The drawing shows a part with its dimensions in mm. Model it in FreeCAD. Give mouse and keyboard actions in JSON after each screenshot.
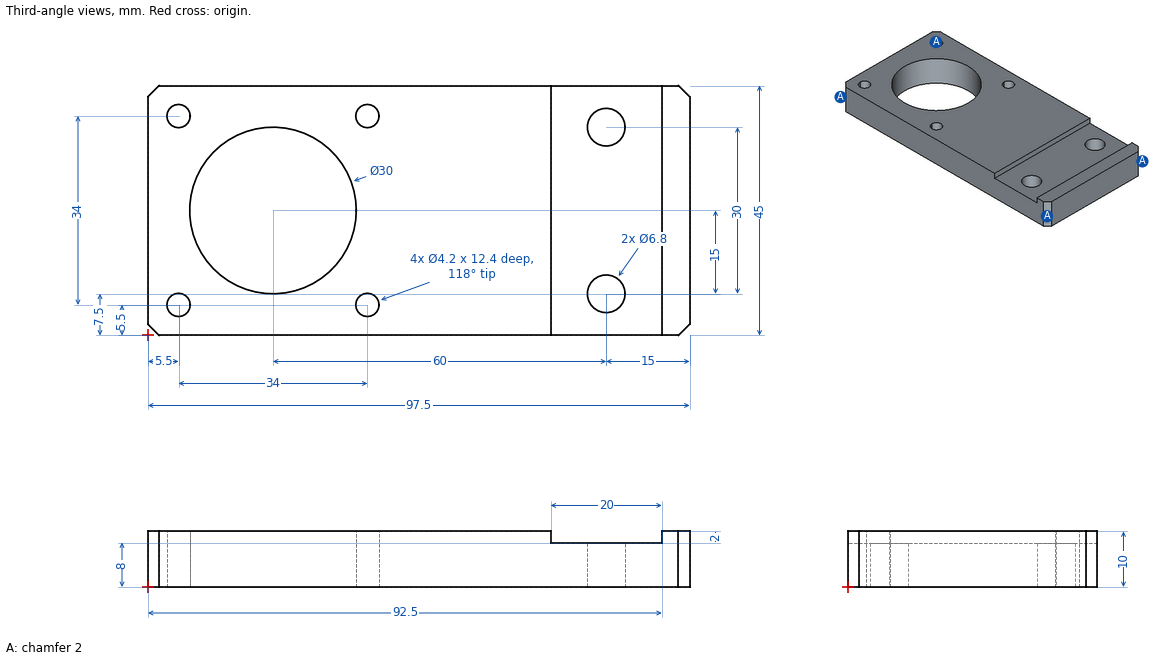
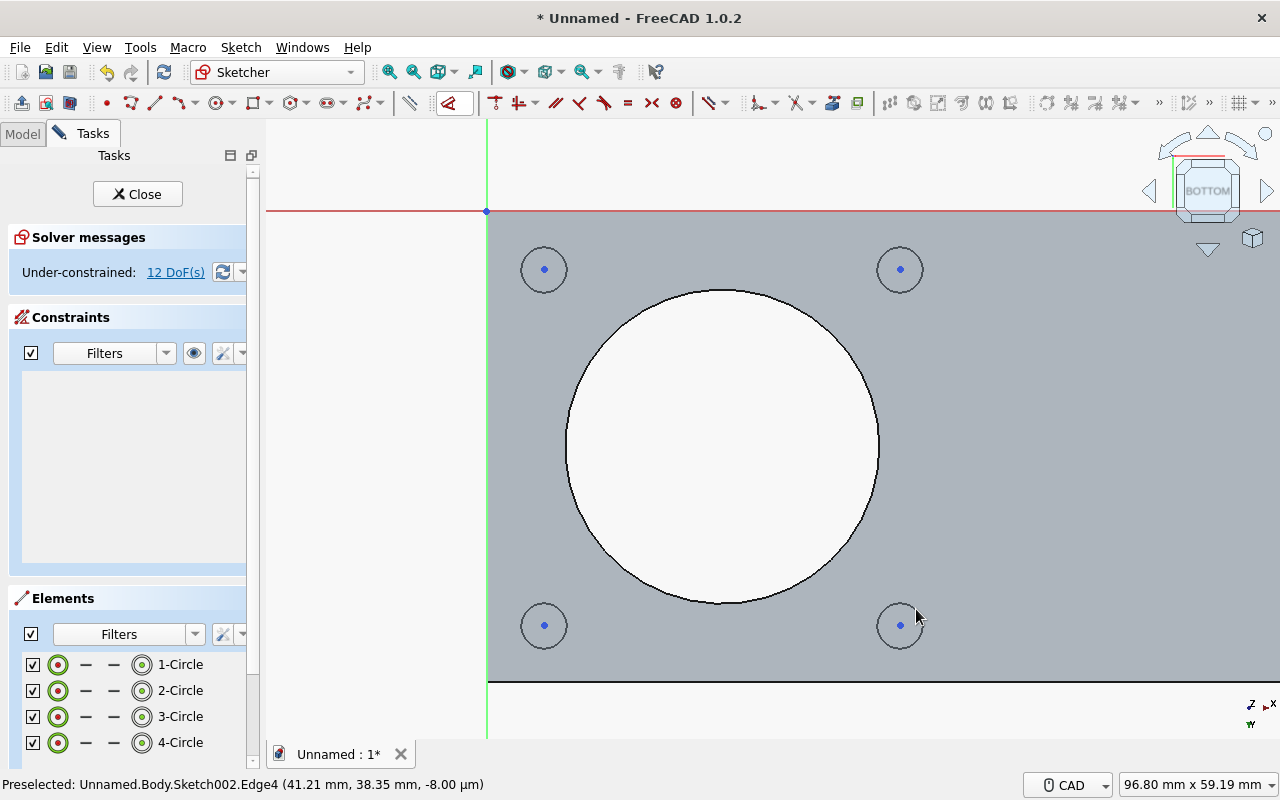
{"action": "left_click", "coordinate": [916, 254]}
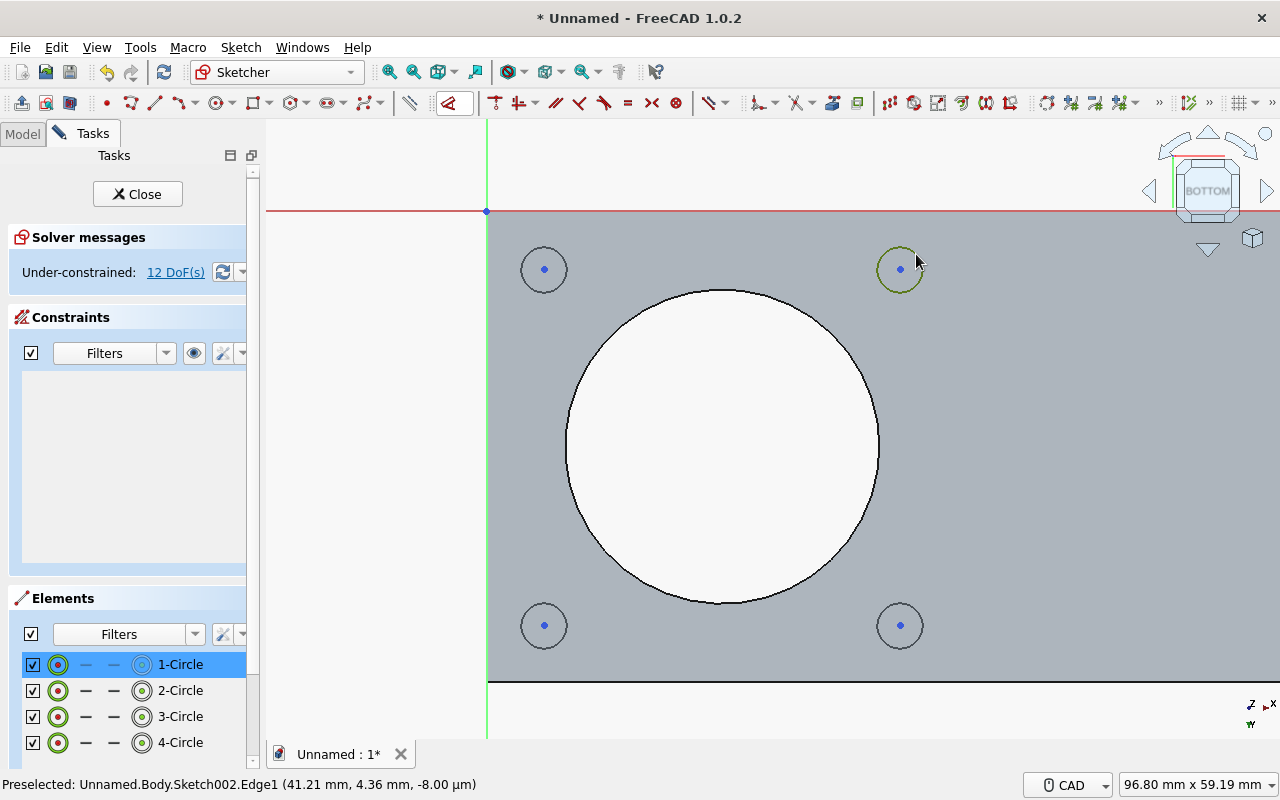
{"action": "left_click", "coordinate": [560, 254]}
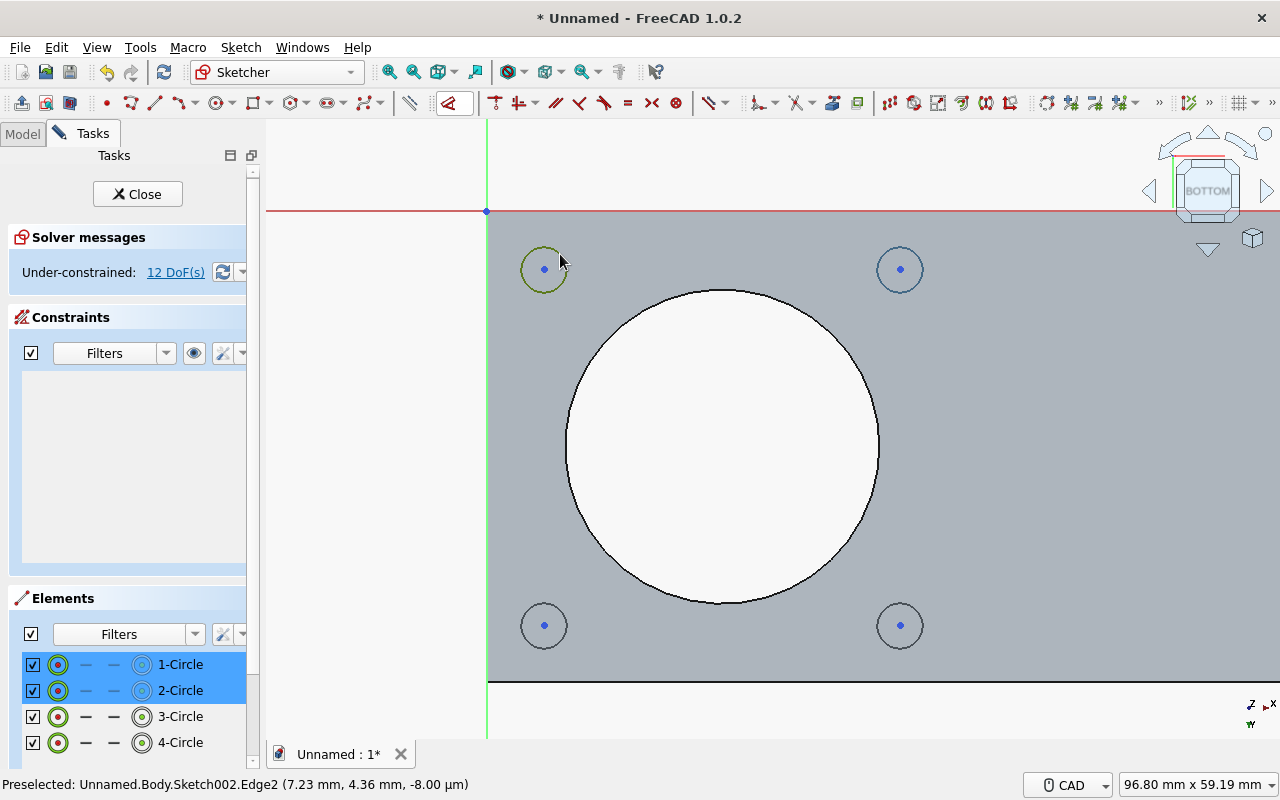
{"action": "left_click", "coordinate": [560, 610]}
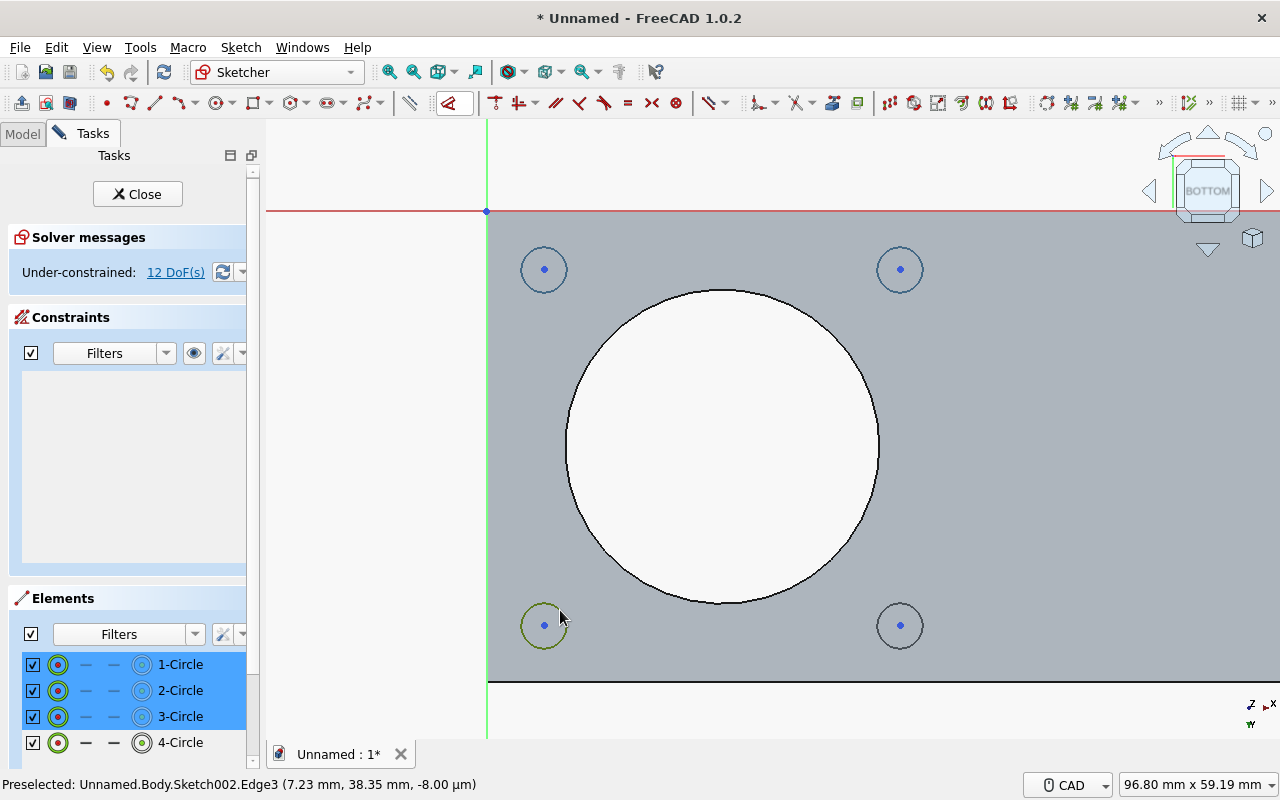
{"action": "left_click", "coordinate": [916, 610]}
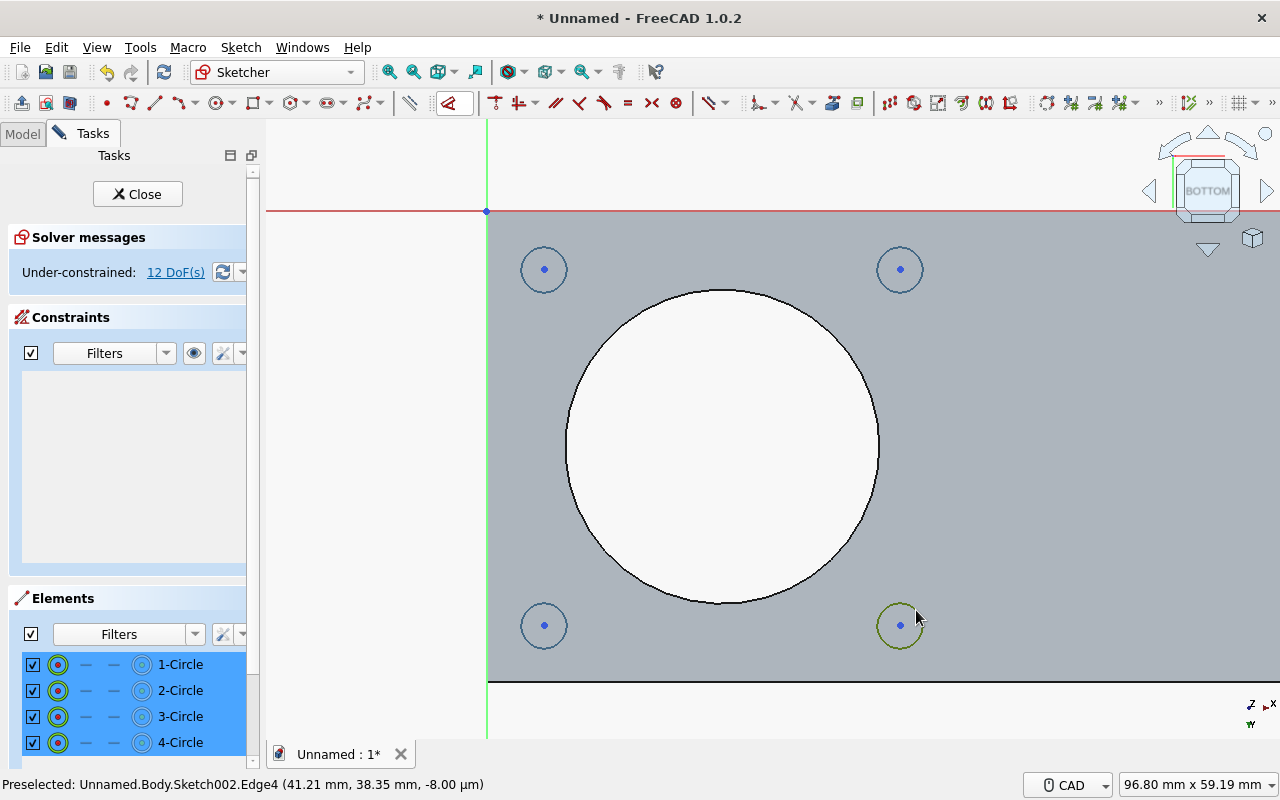
{"action": "key", "text": "e"}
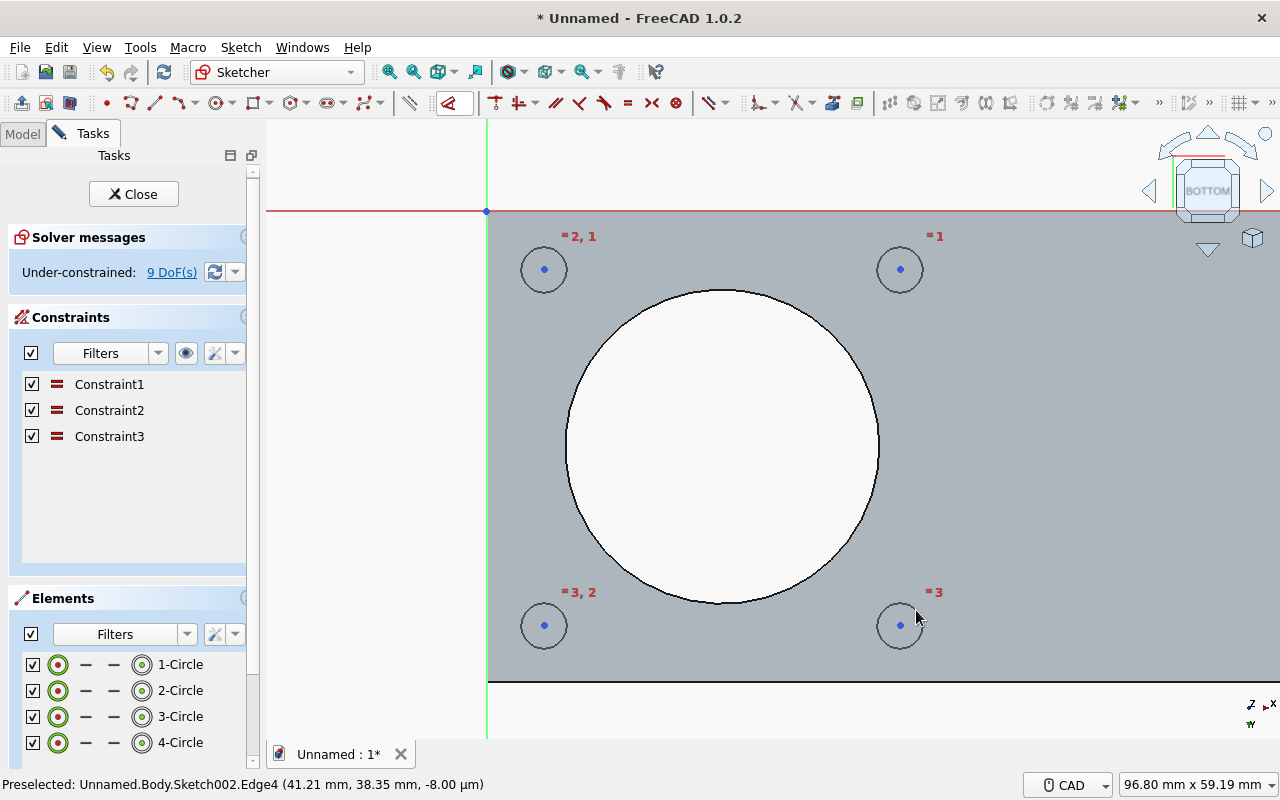
{"action": "left_click", "coordinate": [900, 270]}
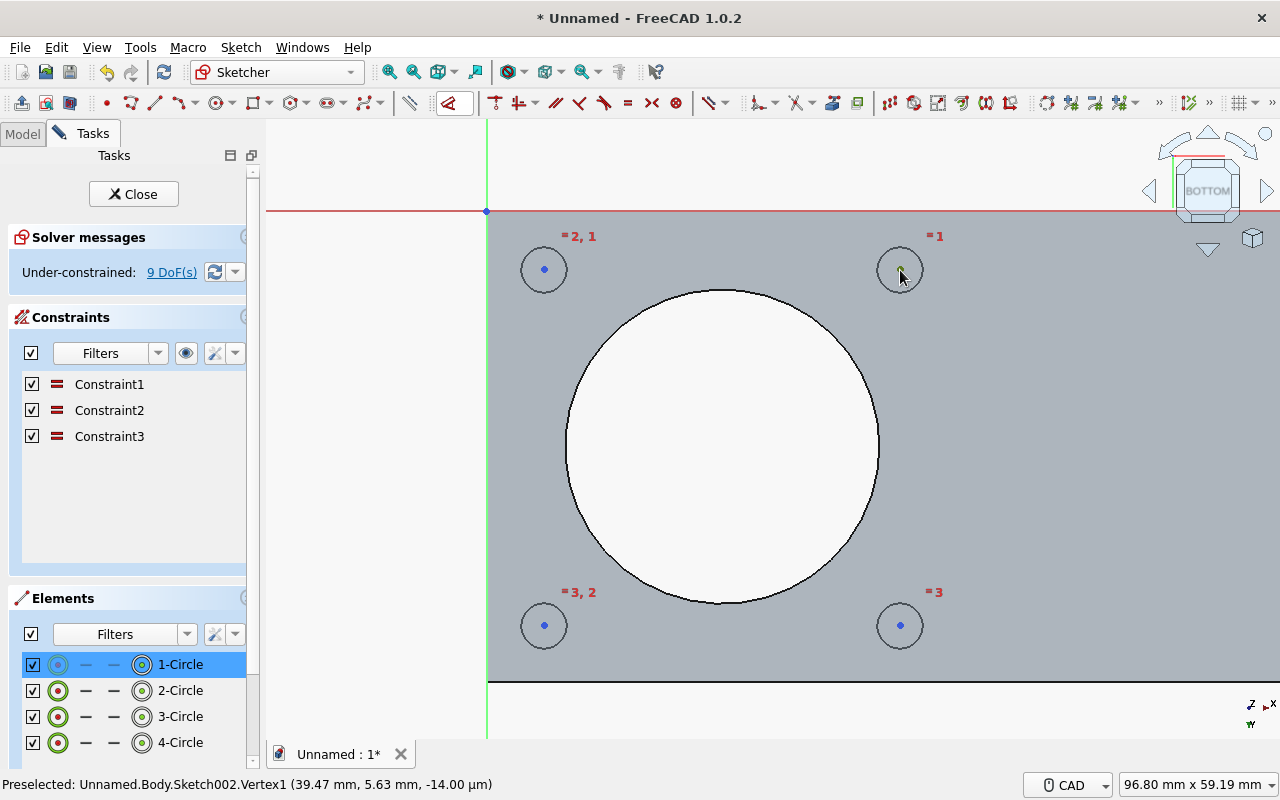
{"action": "left_click", "coordinate": [544, 270]}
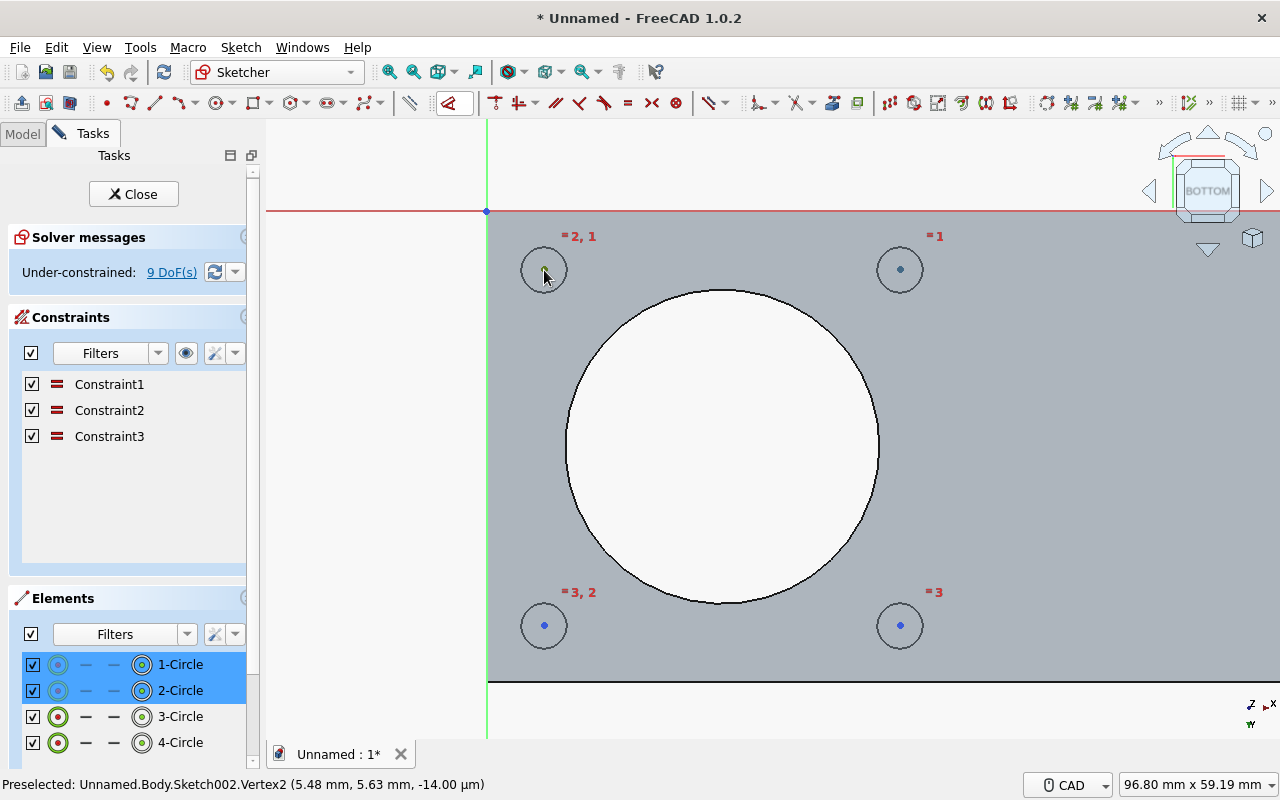
{"action": "key", "text": "h"}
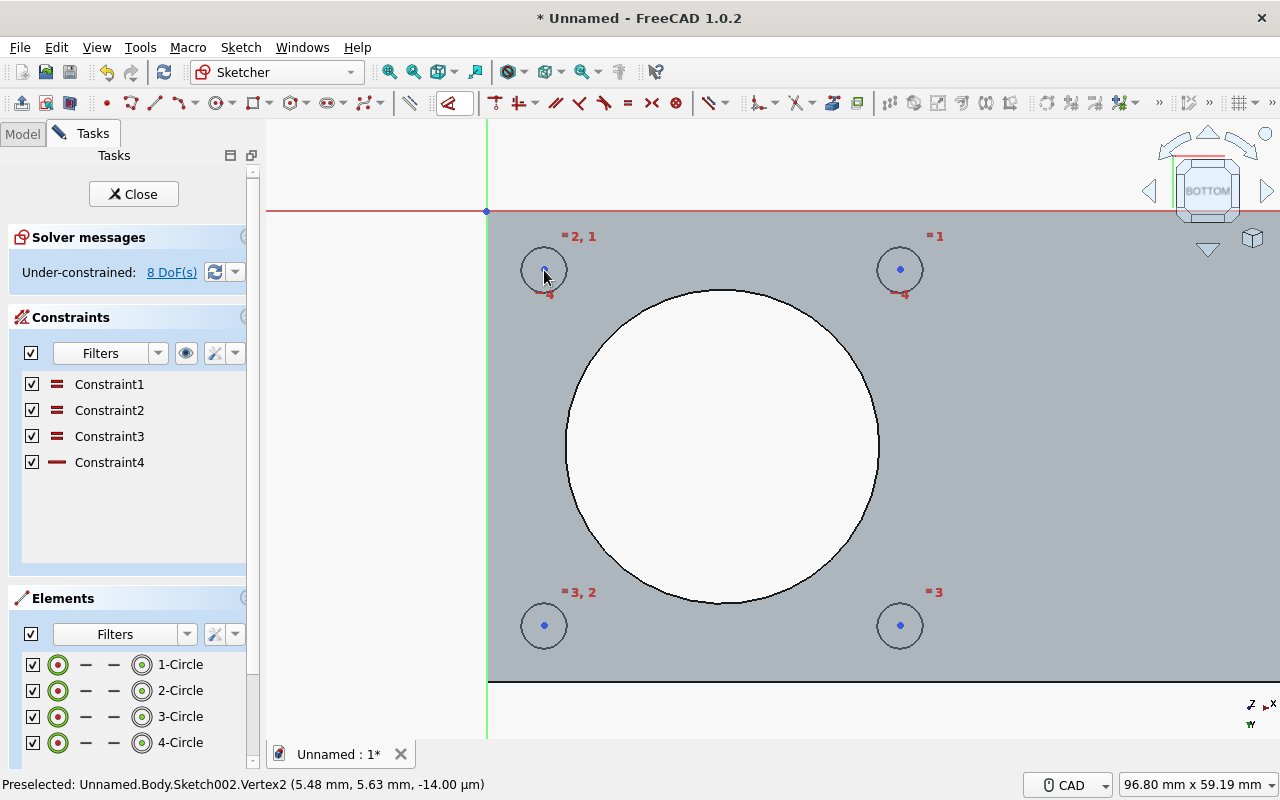
{"action": "left_click", "coordinate": [544, 270]}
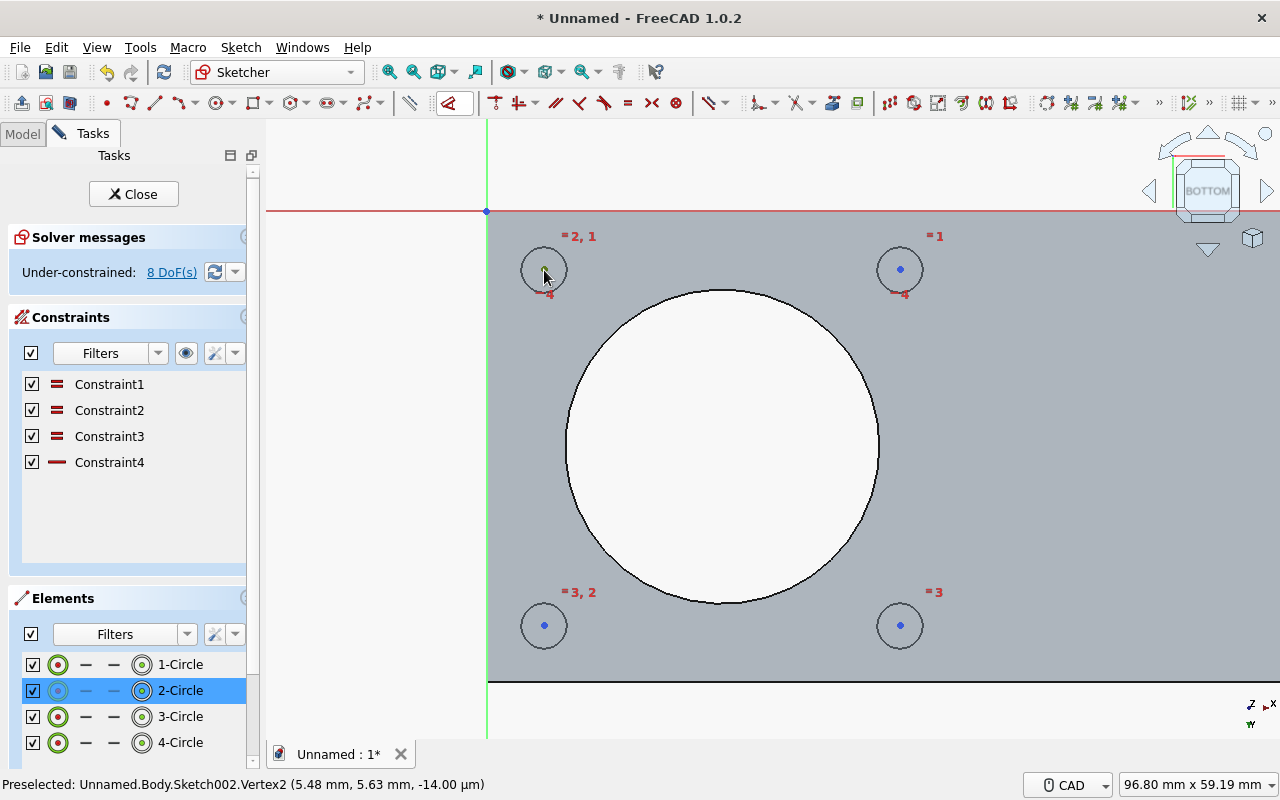
{"action": "left_click", "coordinate": [544, 626]}